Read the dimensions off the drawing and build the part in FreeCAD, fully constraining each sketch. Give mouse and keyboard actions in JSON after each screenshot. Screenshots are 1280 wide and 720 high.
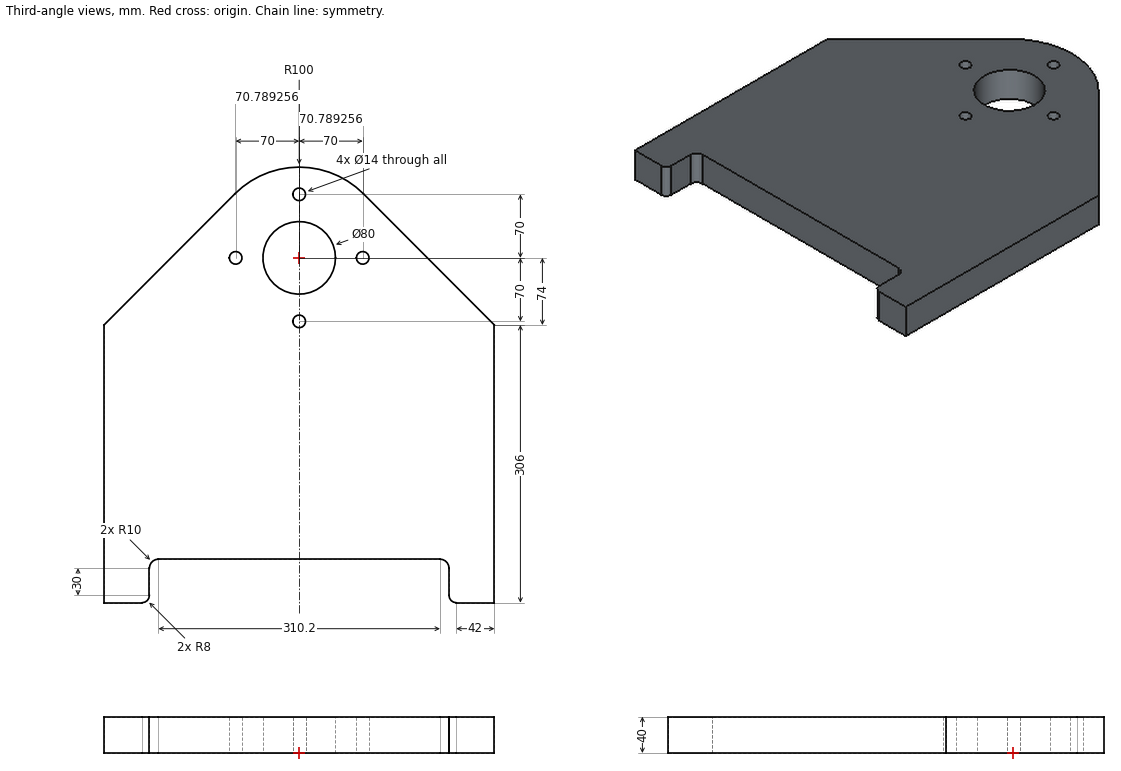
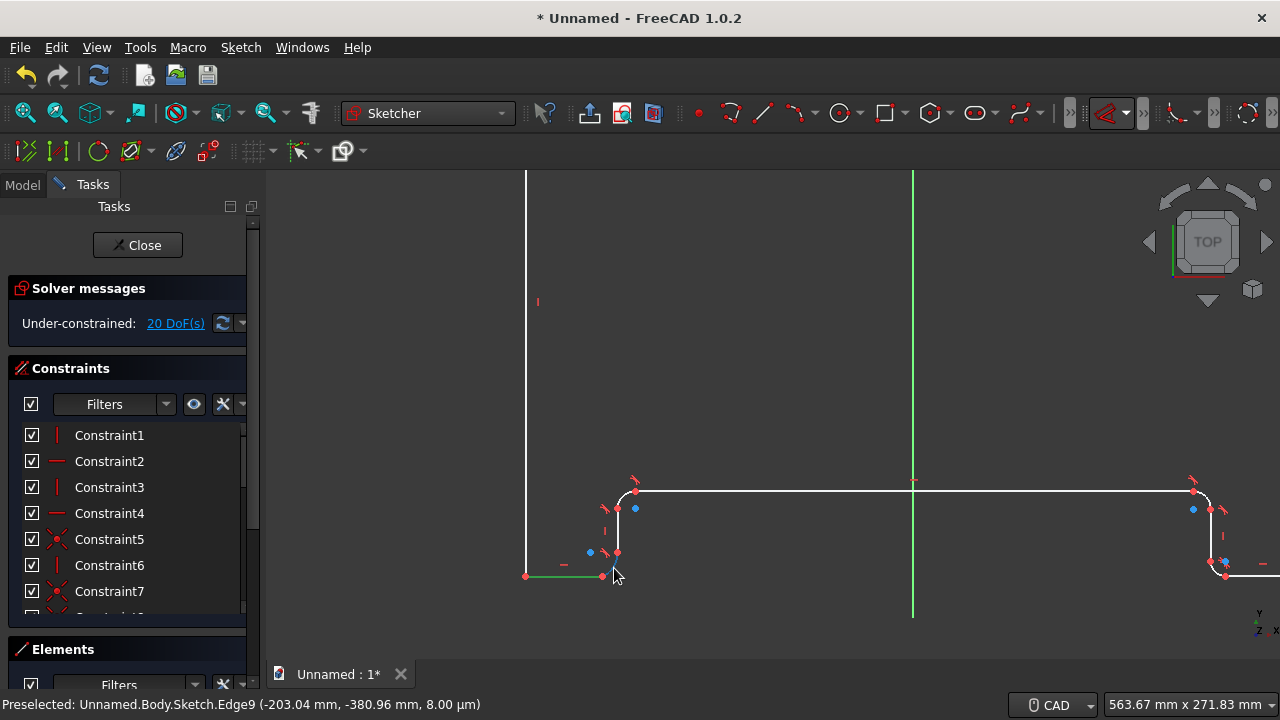
{"action": "left_click", "coordinate": [613, 567]}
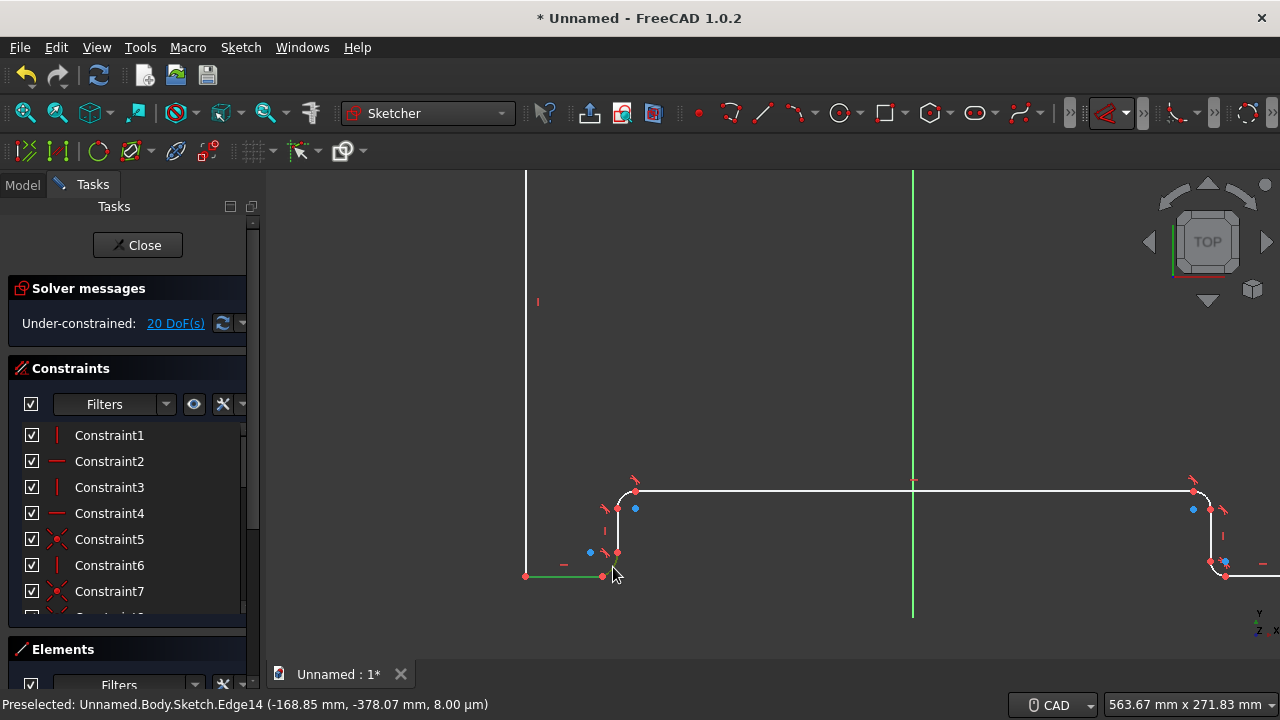
{"action": "key", "text": "t"}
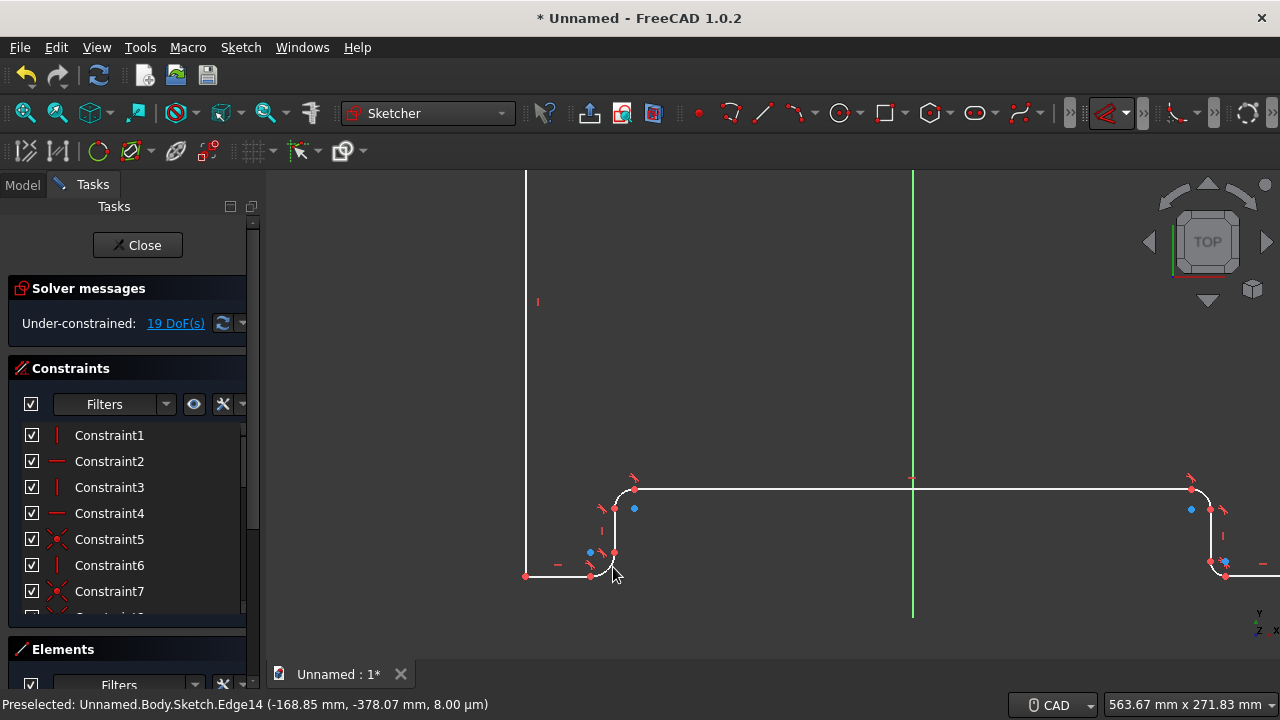
{"action": "scroll", "coordinate": [583, 572], "scroll_direction": "down", "scroll_amount": 5}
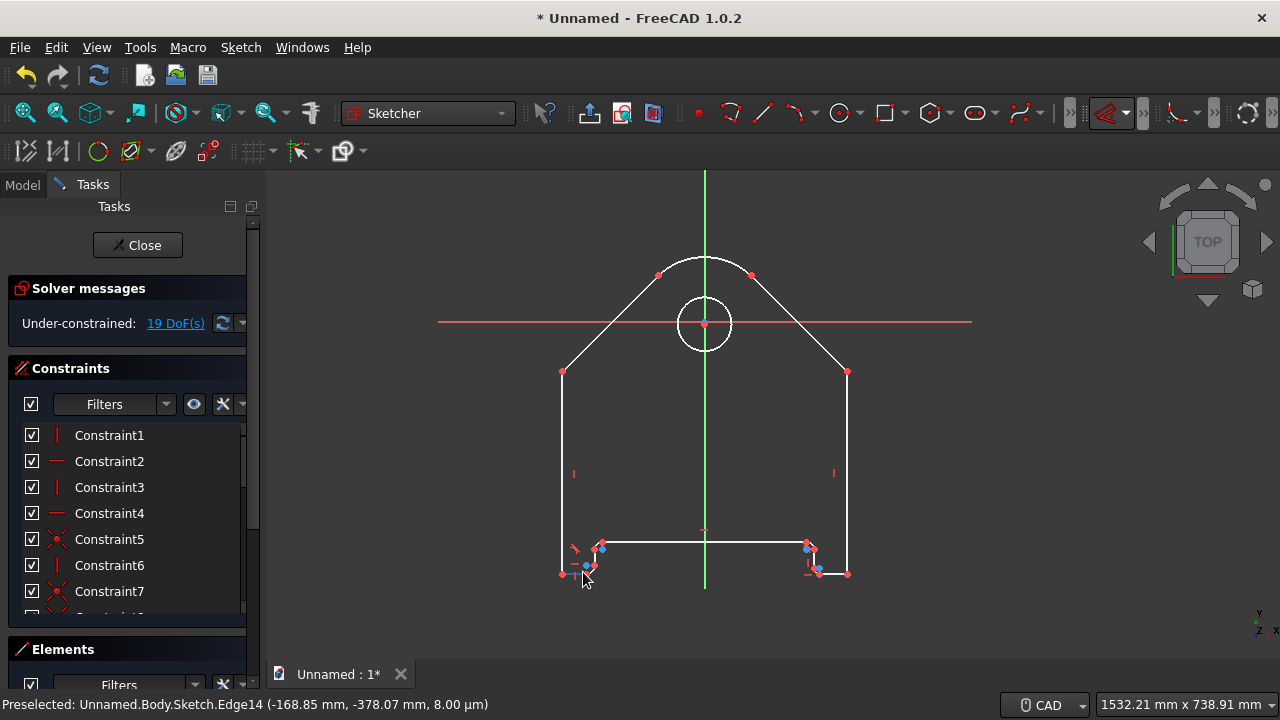
{"action": "scroll", "coordinate": [705, 323], "scroll_direction": "up", "scroll_amount": 10}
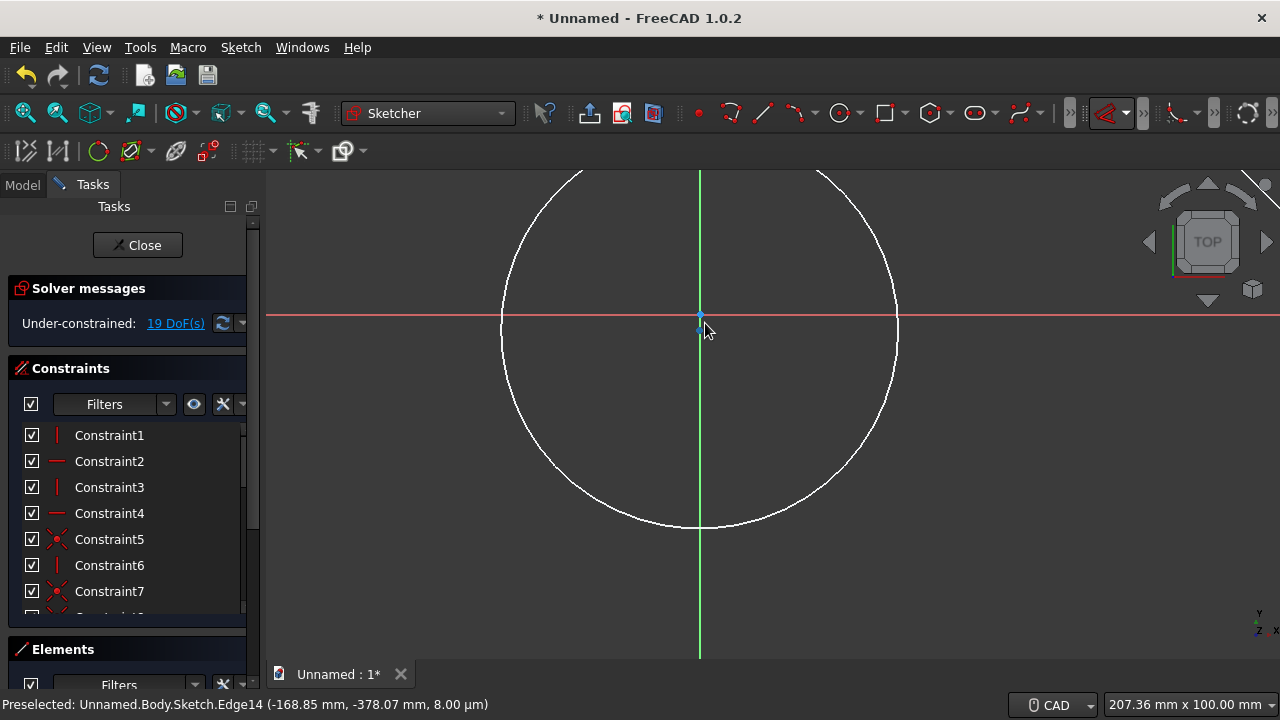
{"action": "left_click_drag", "start_coordinate": [690, 305], "coordinate": [710, 340]}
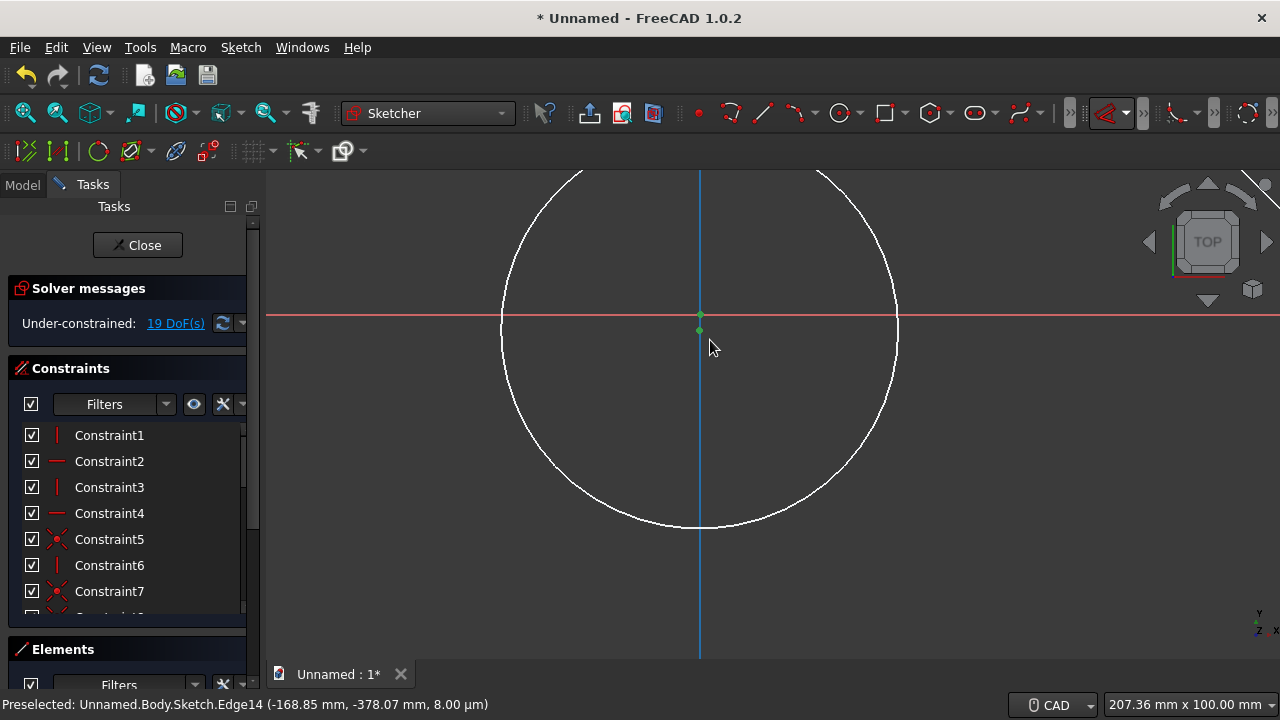
{"action": "key", "text": "c"}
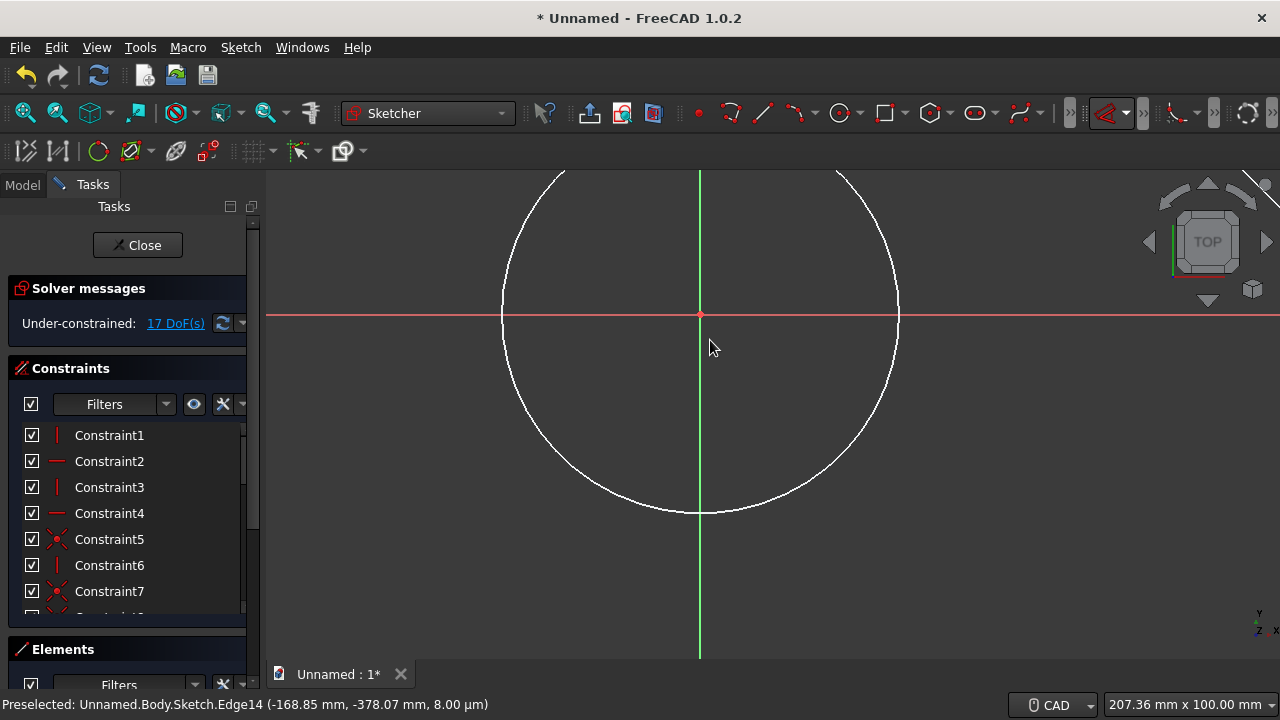
{"action": "scroll", "coordinate": [705, 323], "scroll_direction": "down", "scroll_amount": 10}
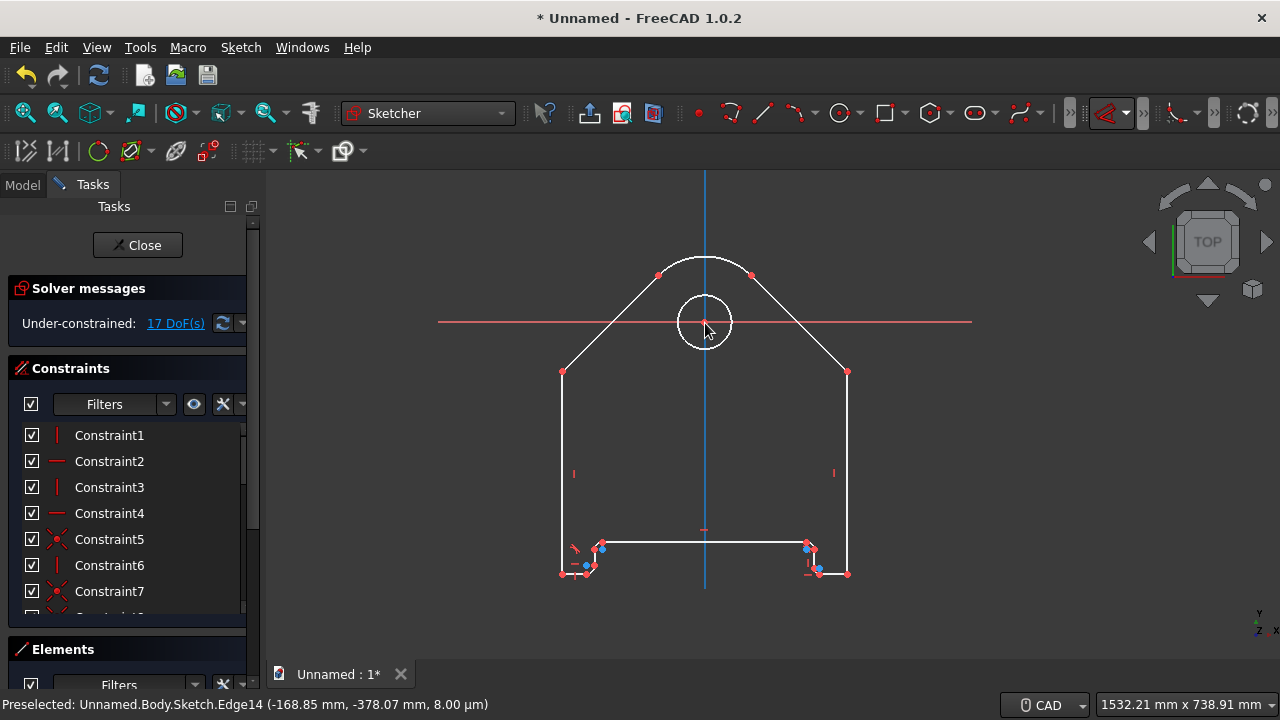
{"action": "scroll", "coordinate": [599, 543], "scroll_direction": "up", "scroll_amount": 8}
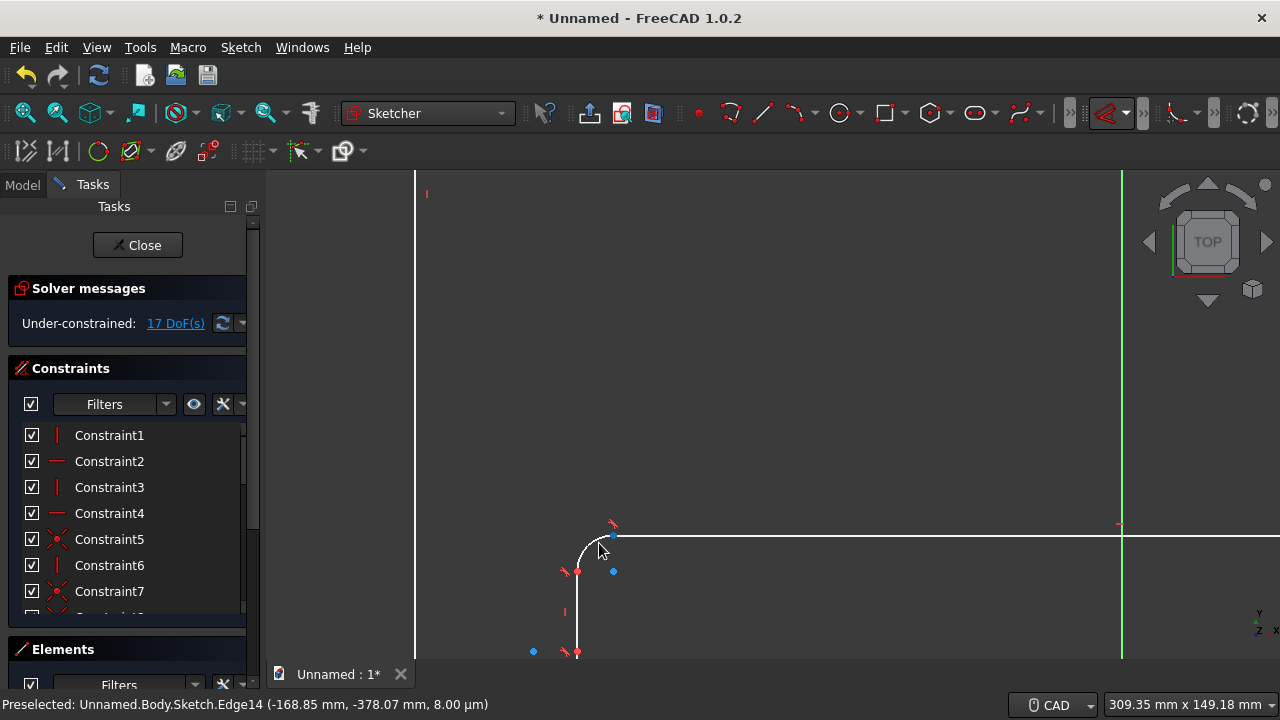
{"action": "left_click", "coordinate": [597, 539]}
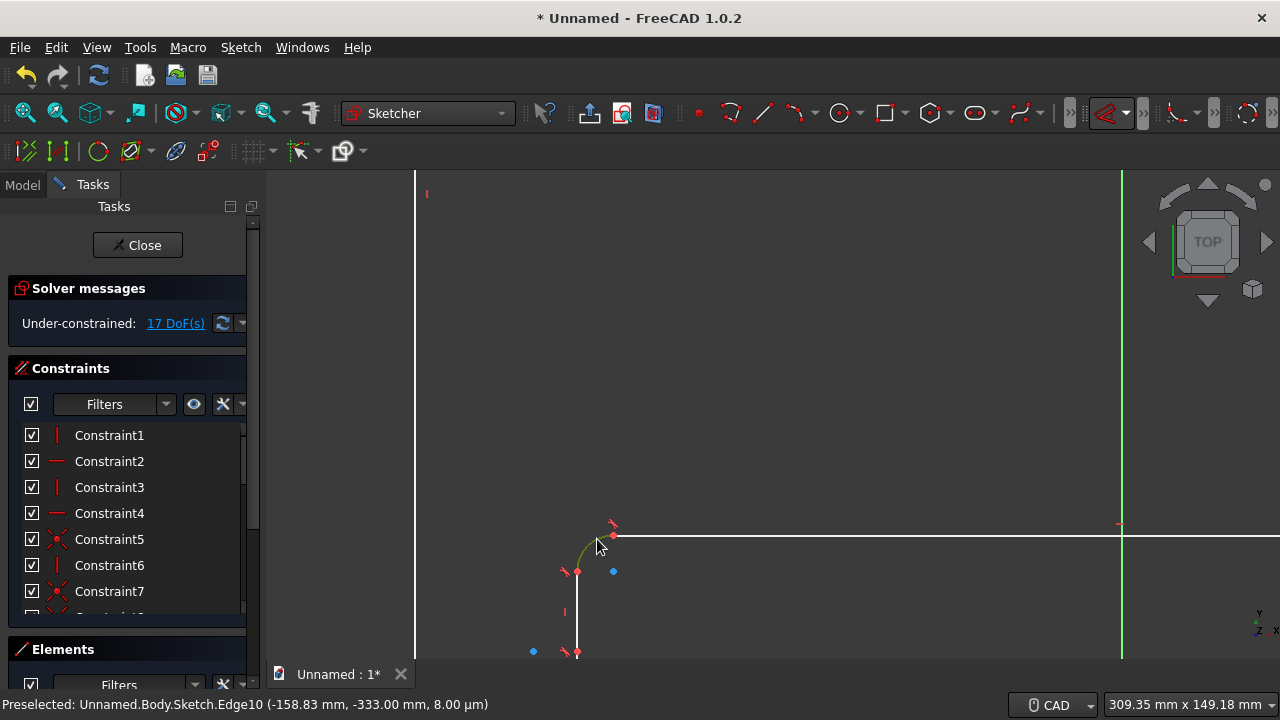
{"action": "scroll", "coordinate": [599, 543], "scroll_direction": "down", "scroll_amount": 8}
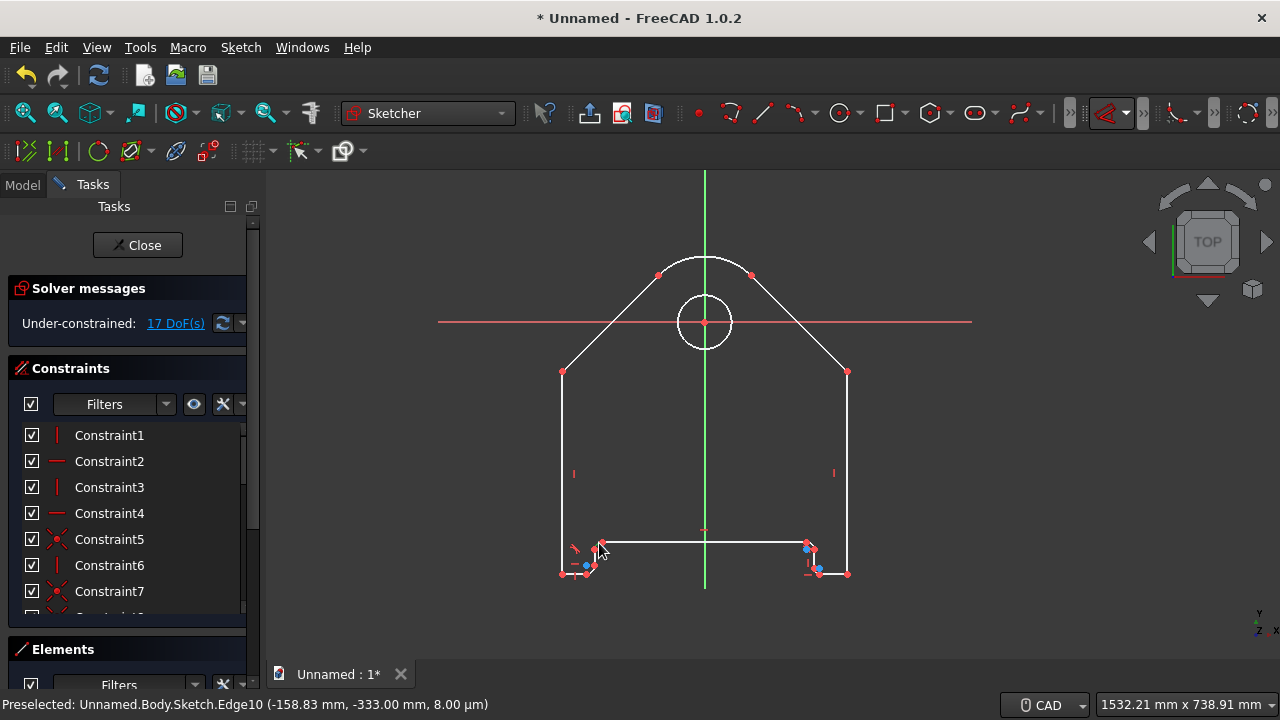
{"action": "scroll", "coordinate": [813, 546], "scroll_direction": "up", "scroll_amount": 8}